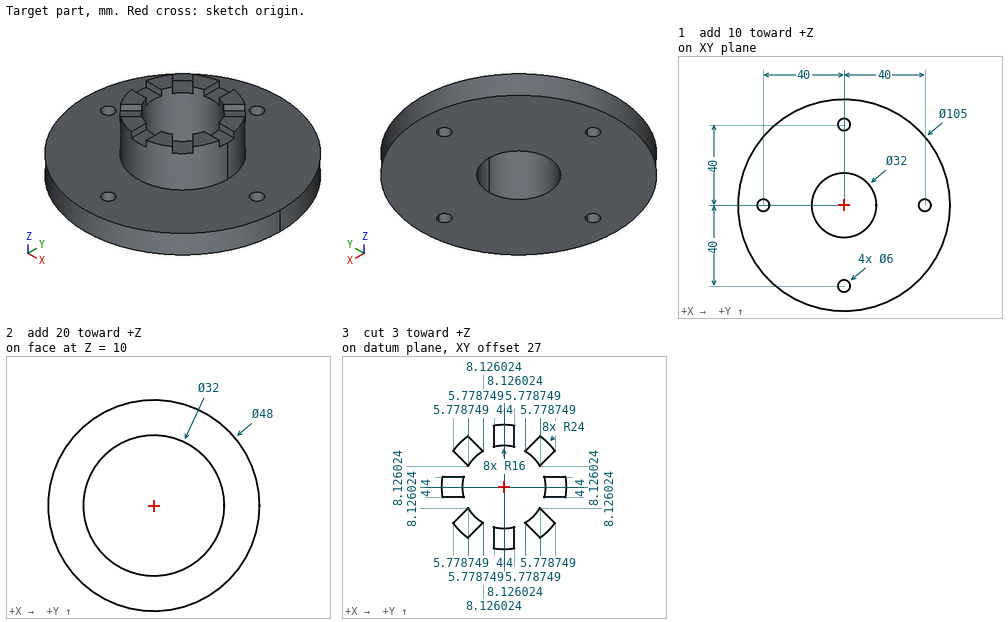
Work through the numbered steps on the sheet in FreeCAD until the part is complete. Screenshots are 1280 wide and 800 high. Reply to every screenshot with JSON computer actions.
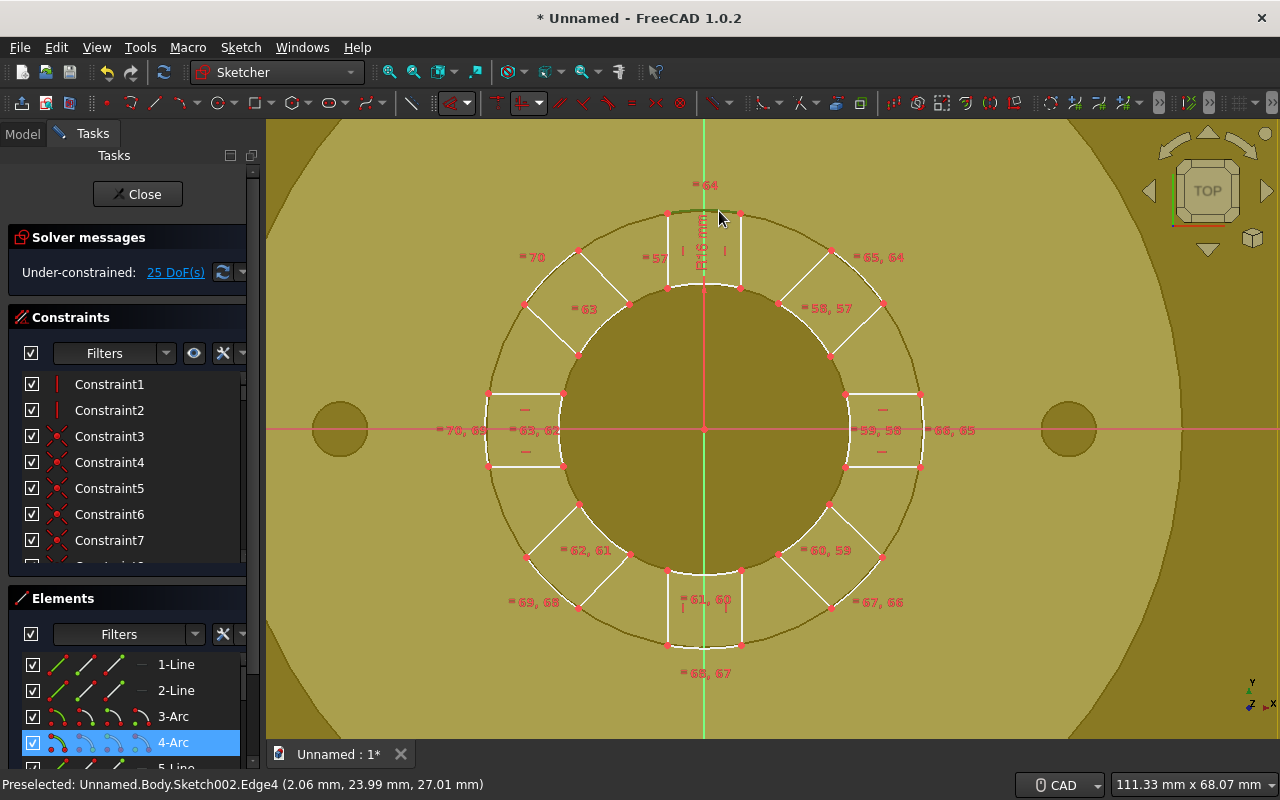
{"action": "key", "text": "k r"}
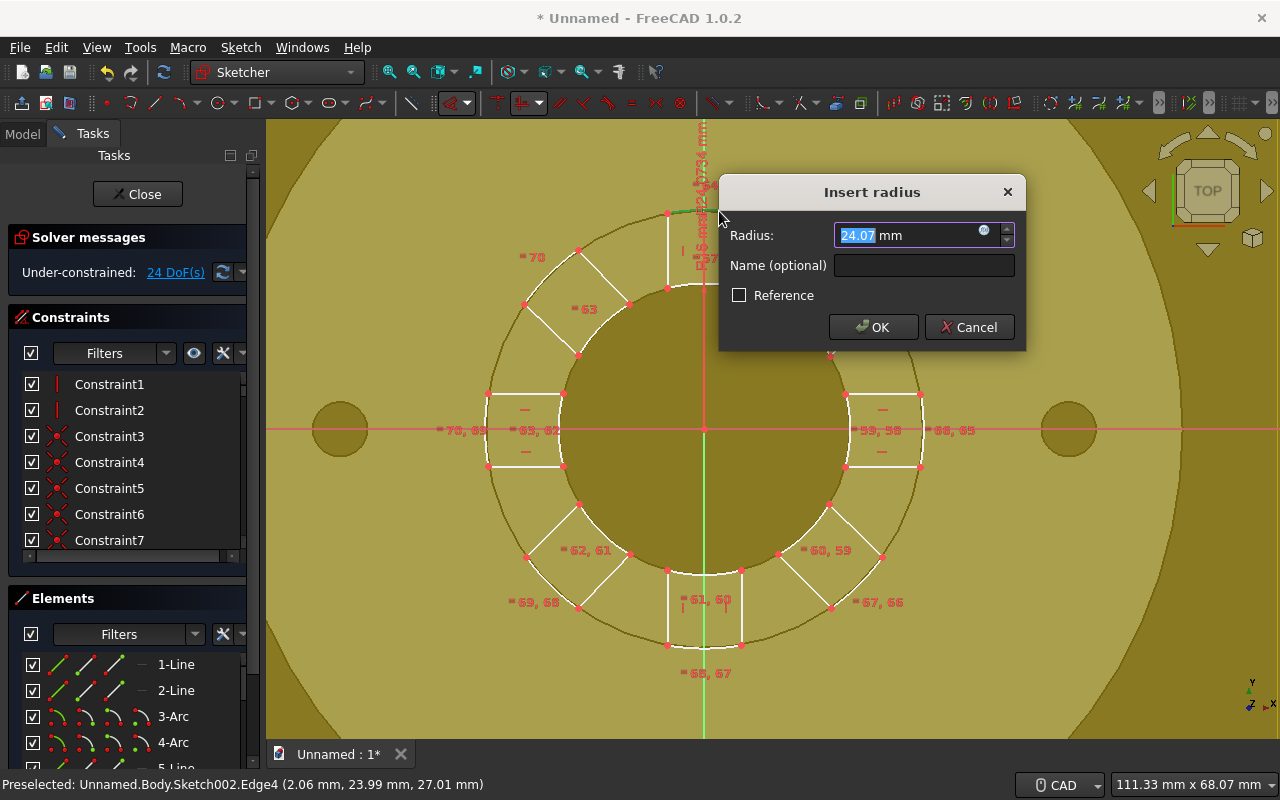
{"action": "type", "text": "24"}
{"action": "key", "text": "Return"}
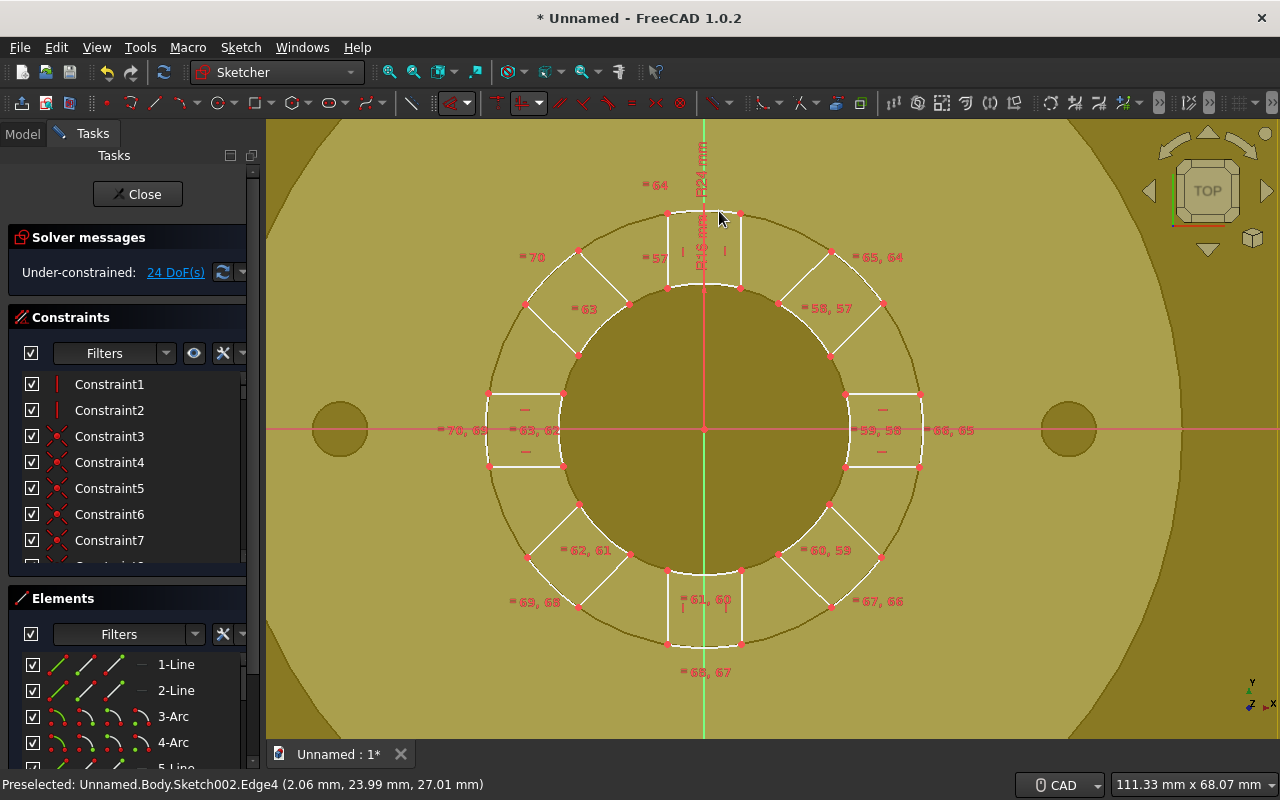
{"action": "left_click", "coordinate": [668, 214]}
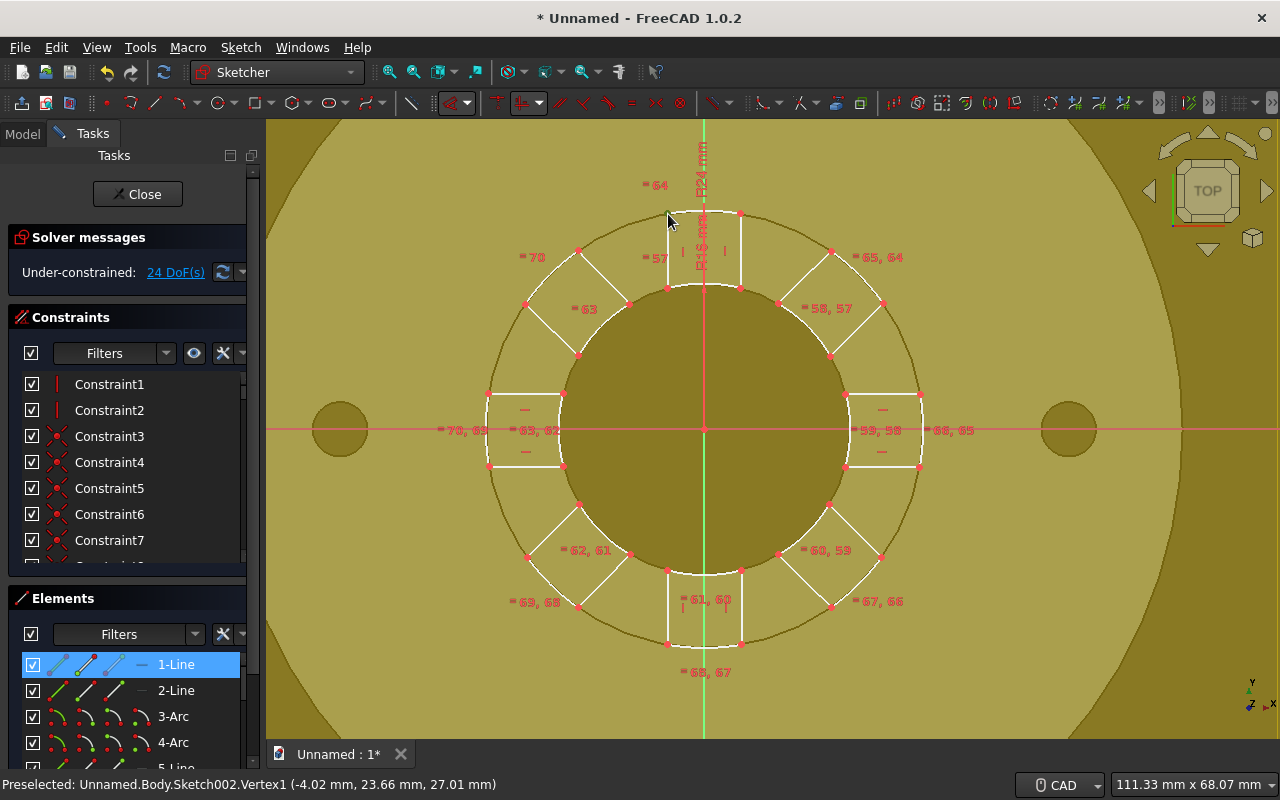
{"action": "left_click", "coordinate": [470, 104]}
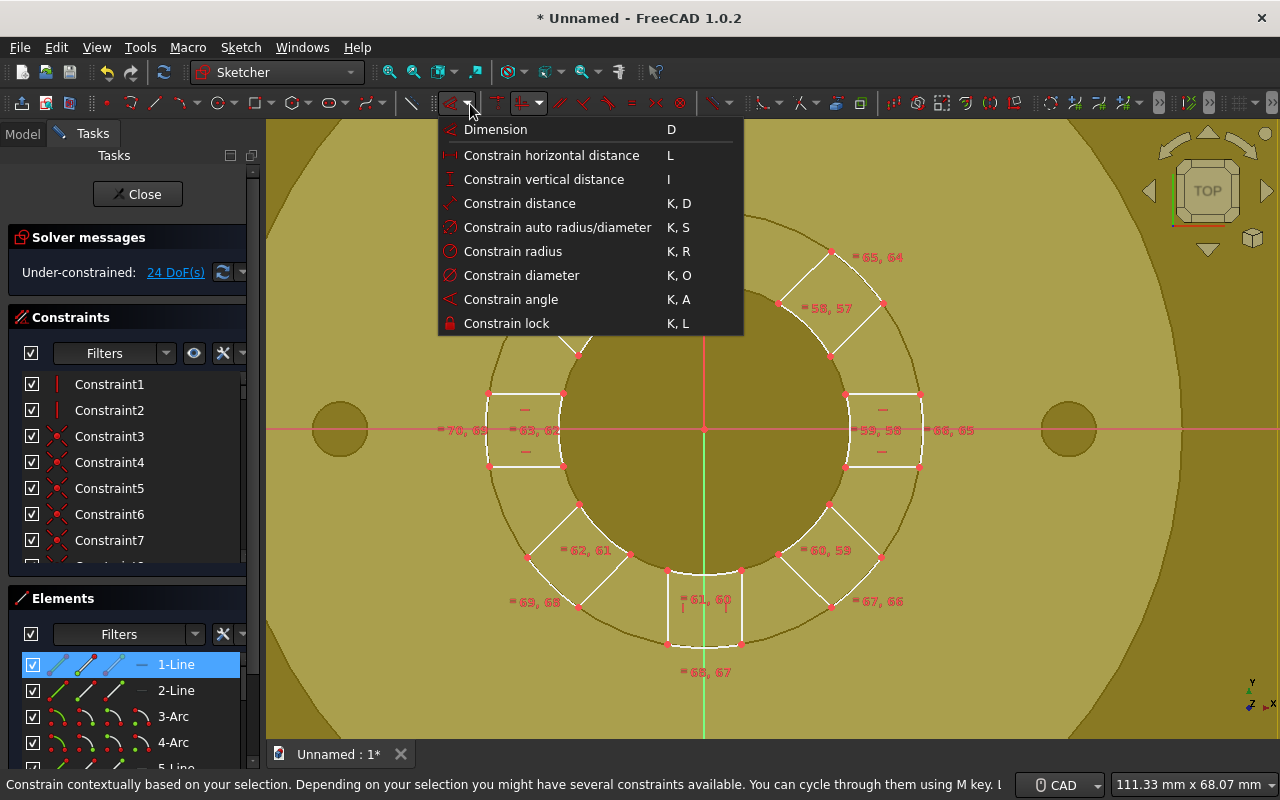
{"action": "left_click", "coordinate": [591, 155]}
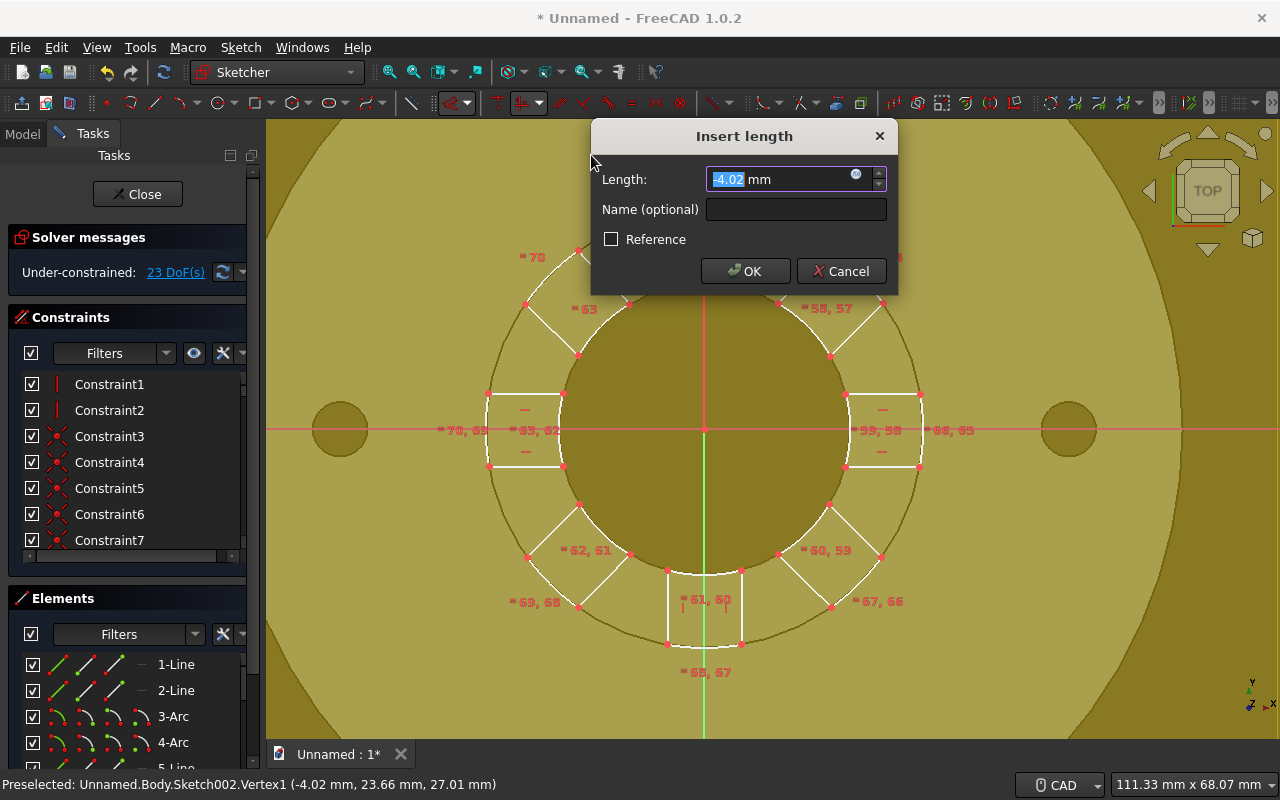
{"action": "type", "text": "-4"}
{"action": "key", "text": "Return"}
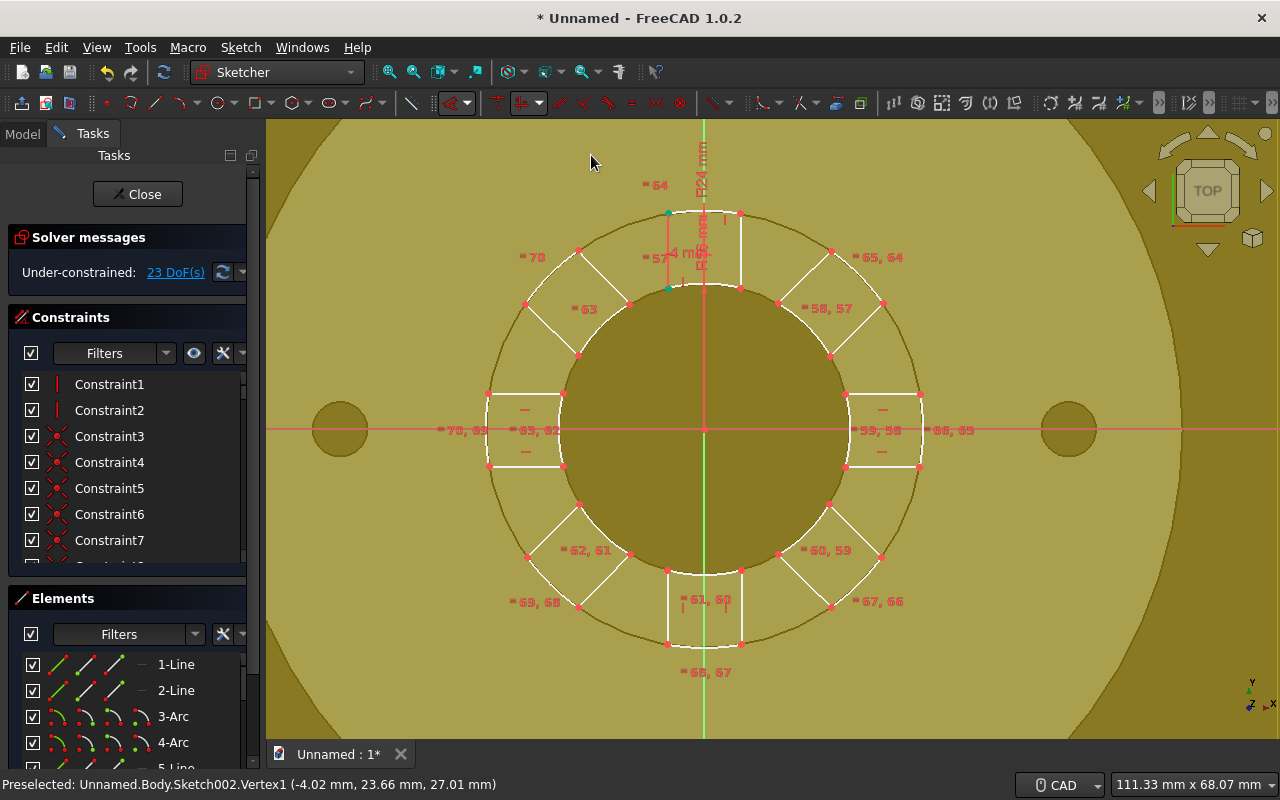
{"action": "left_click", "coordinate": [741, 288]}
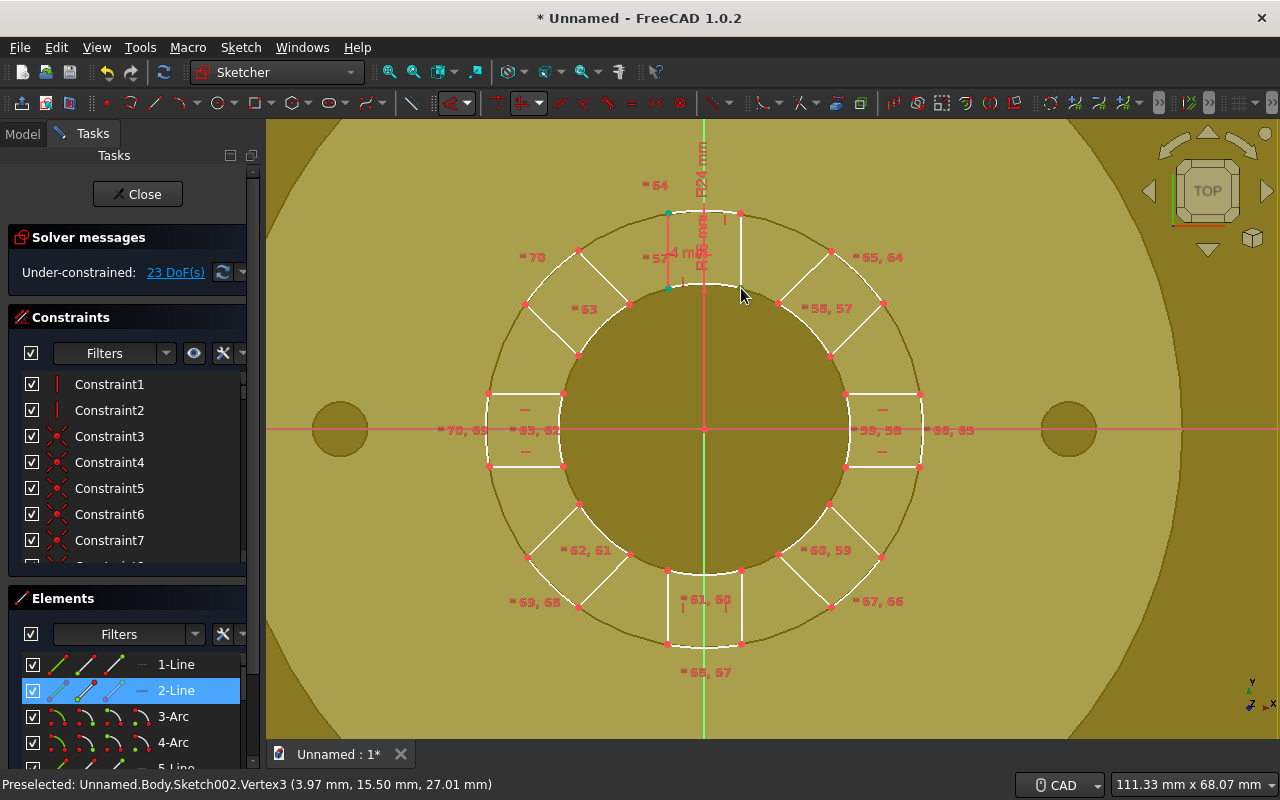
{"action": "key", "text": "l"}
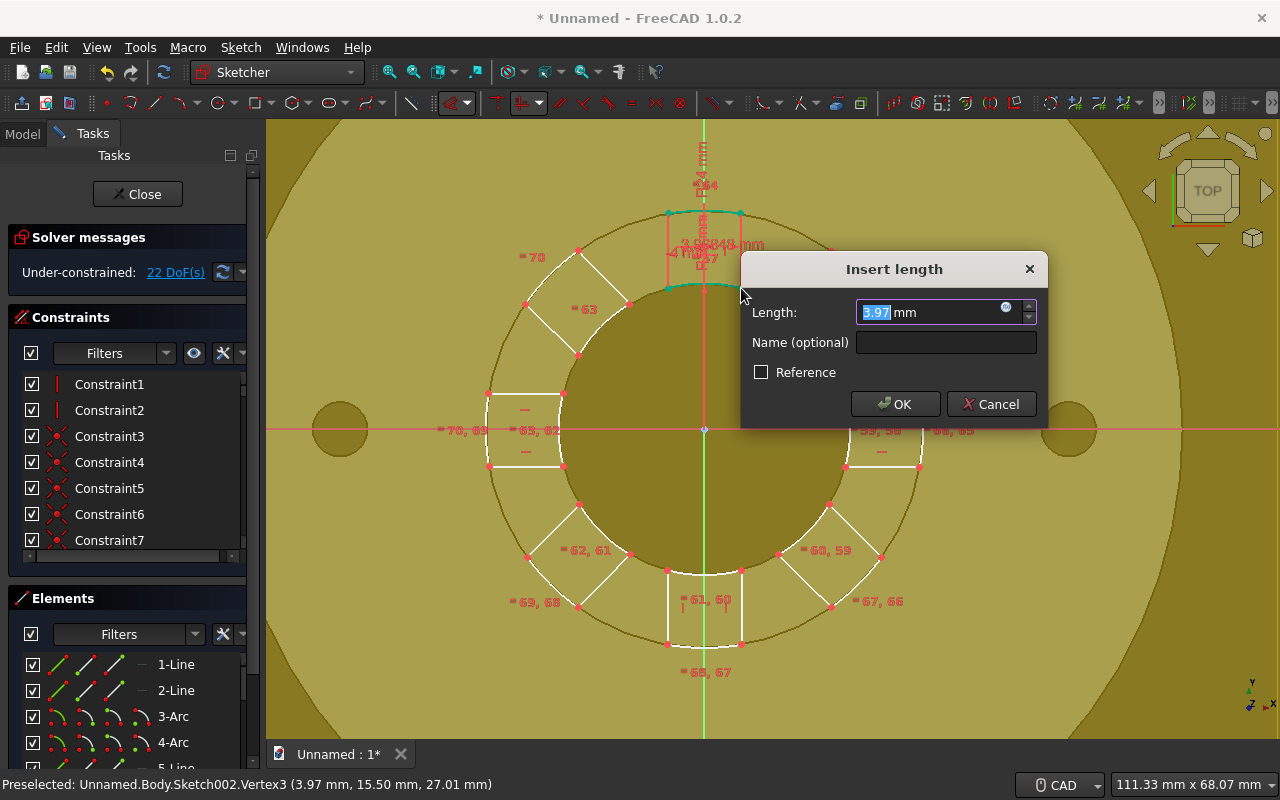
{"action": "type", "text": "4"}
{"action": "key", "text": "Return"}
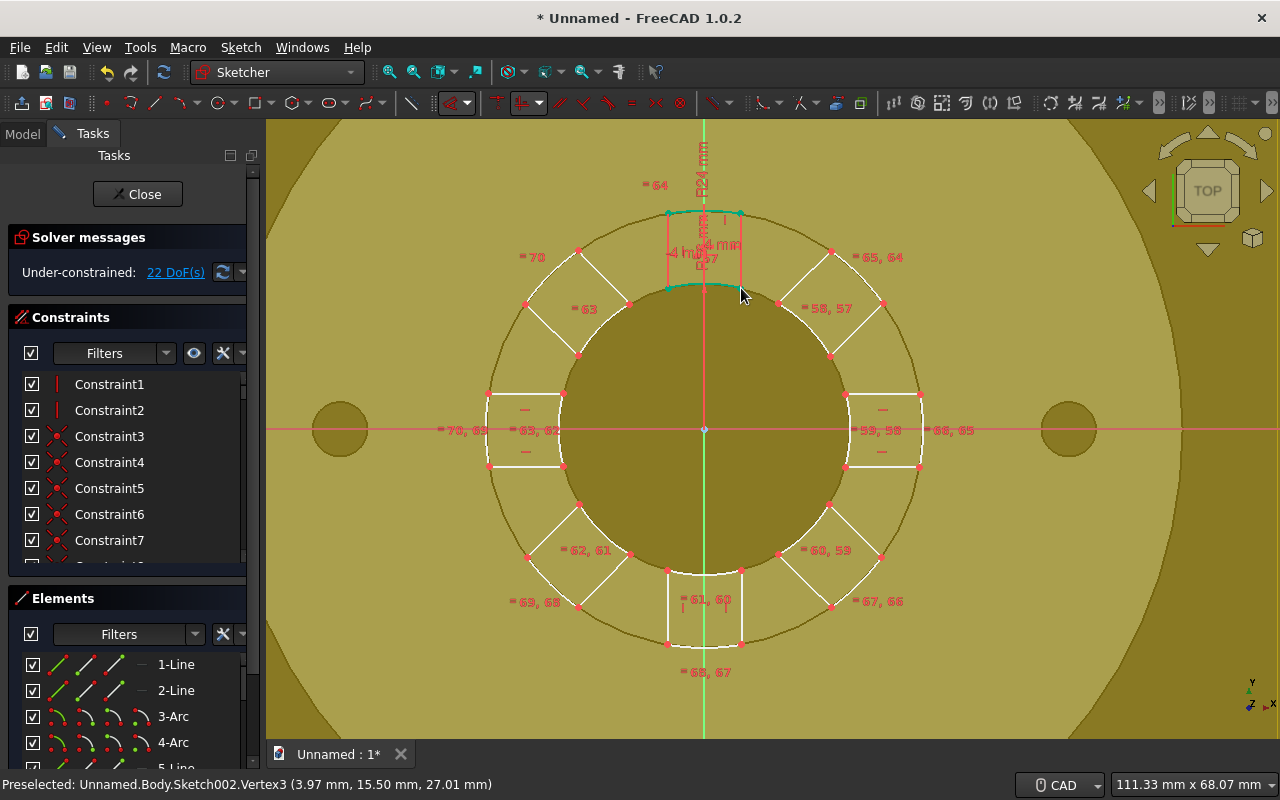
{"action": "left_click", "coordinate": [920, 394]}